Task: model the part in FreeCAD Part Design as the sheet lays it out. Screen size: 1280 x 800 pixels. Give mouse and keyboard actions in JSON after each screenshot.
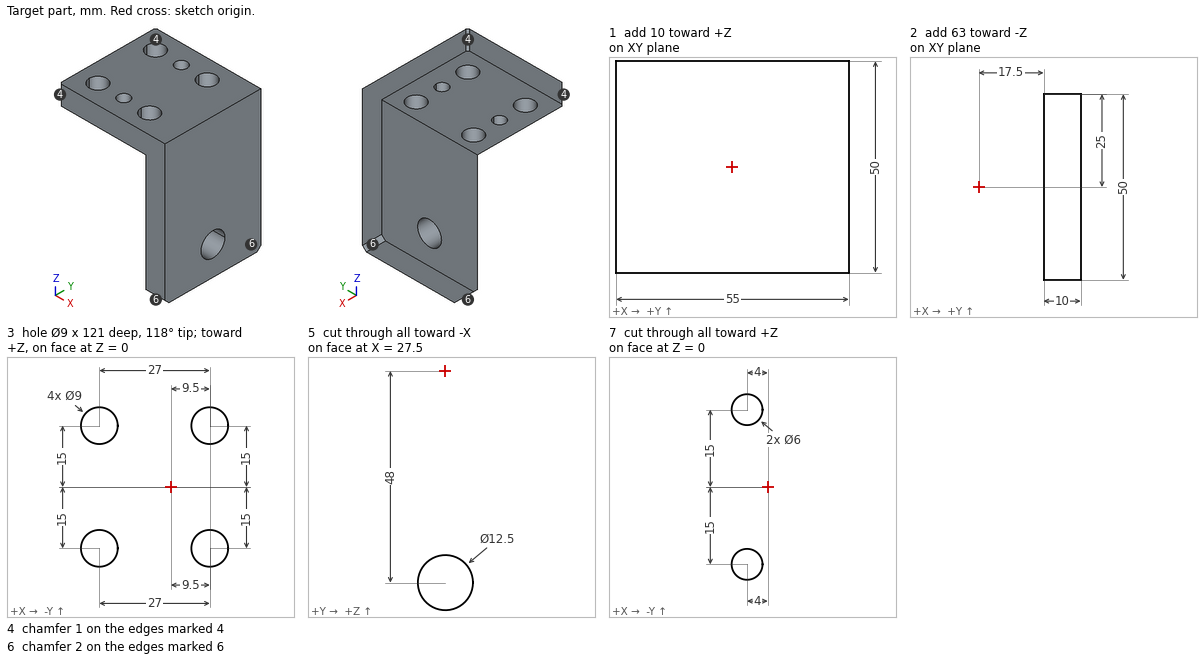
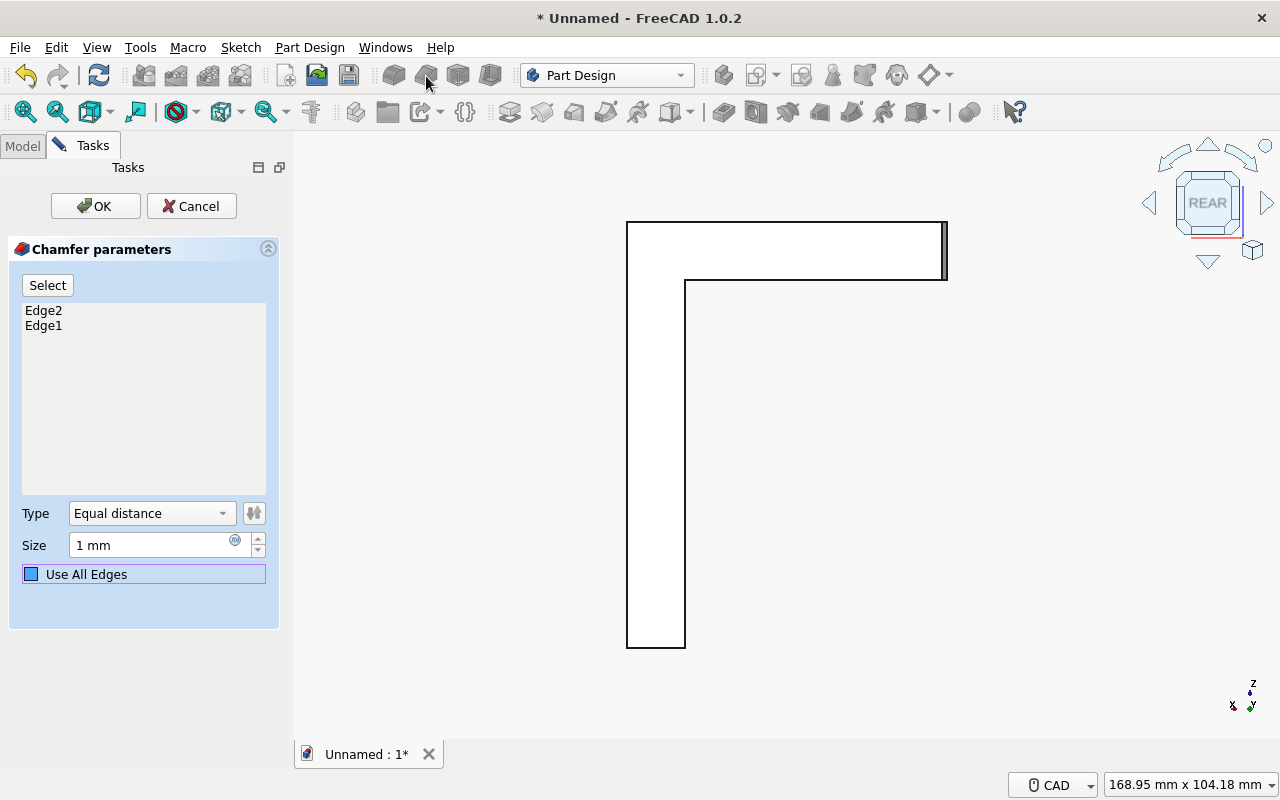
{"action": "left_click", "coordinate": [96, 206]}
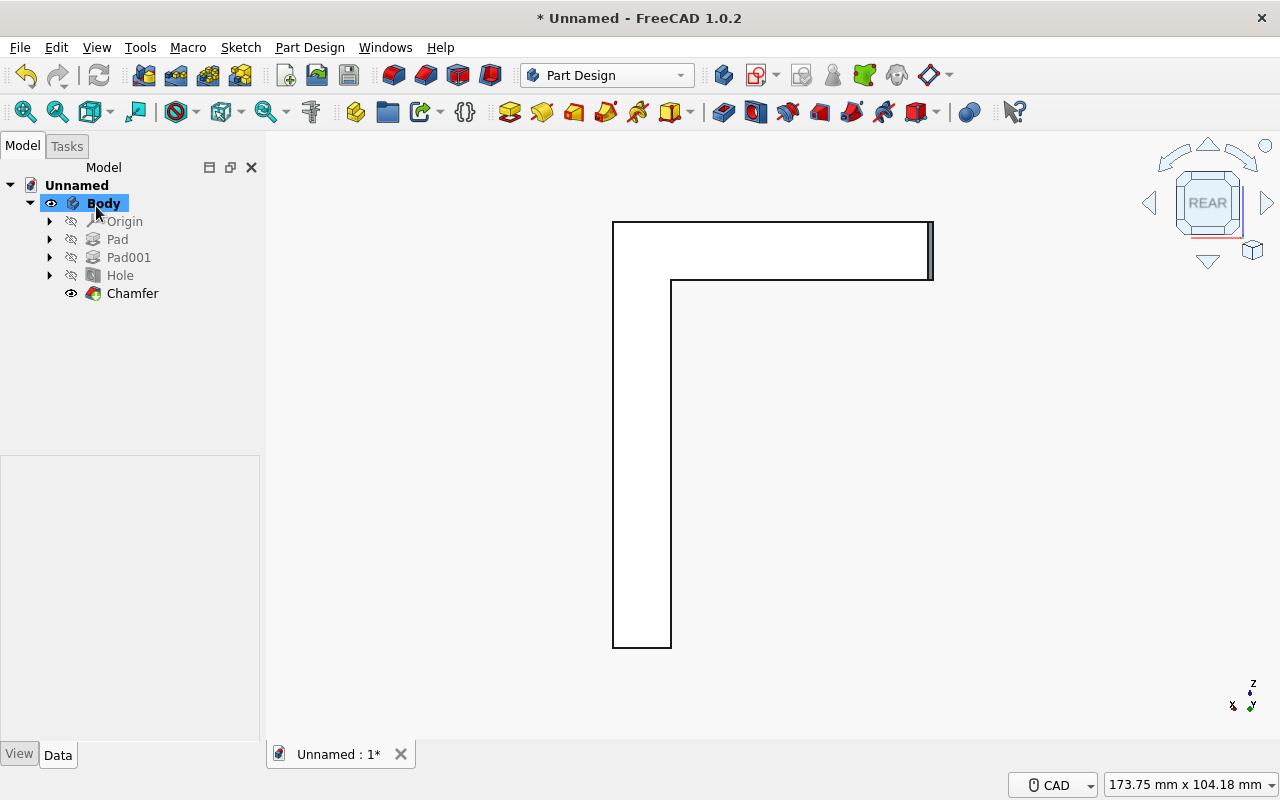
{"action": "key", "text": "0"}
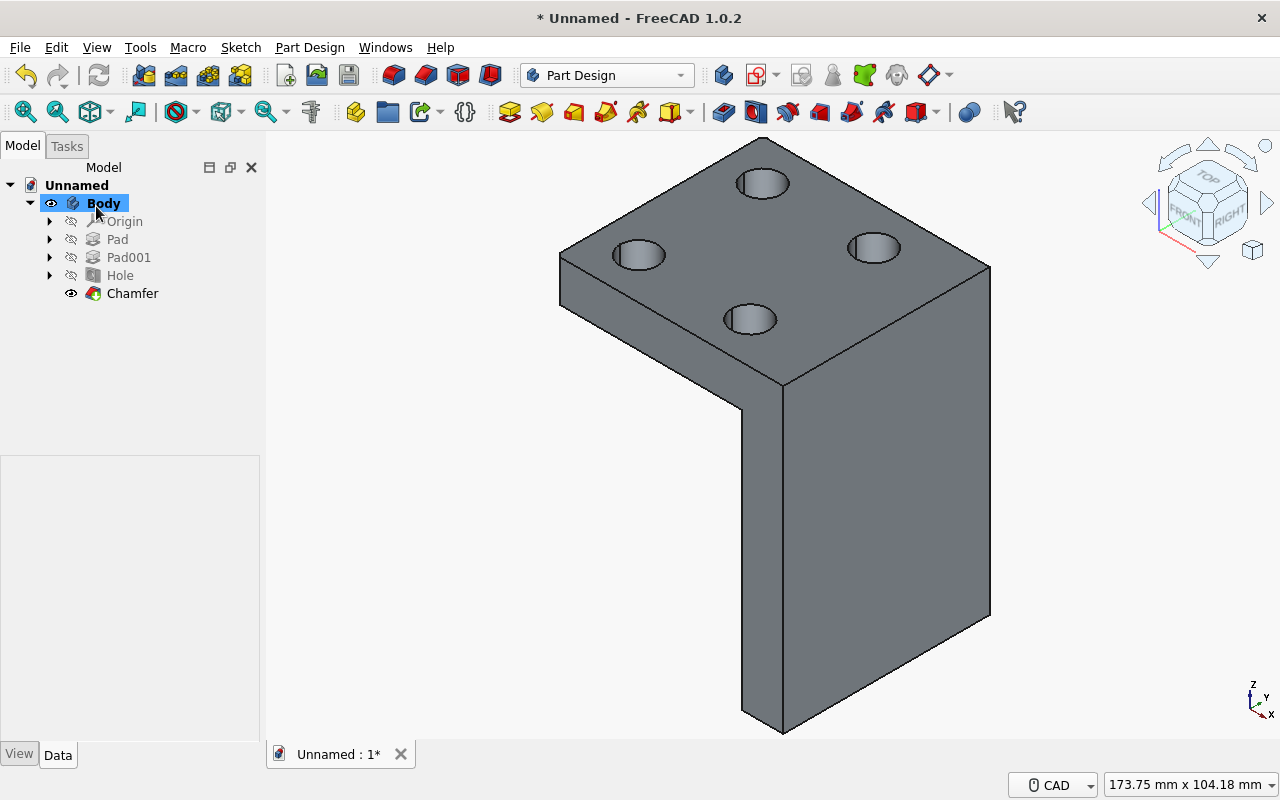
{"action": "left_click", "coordinate": [886, 450]}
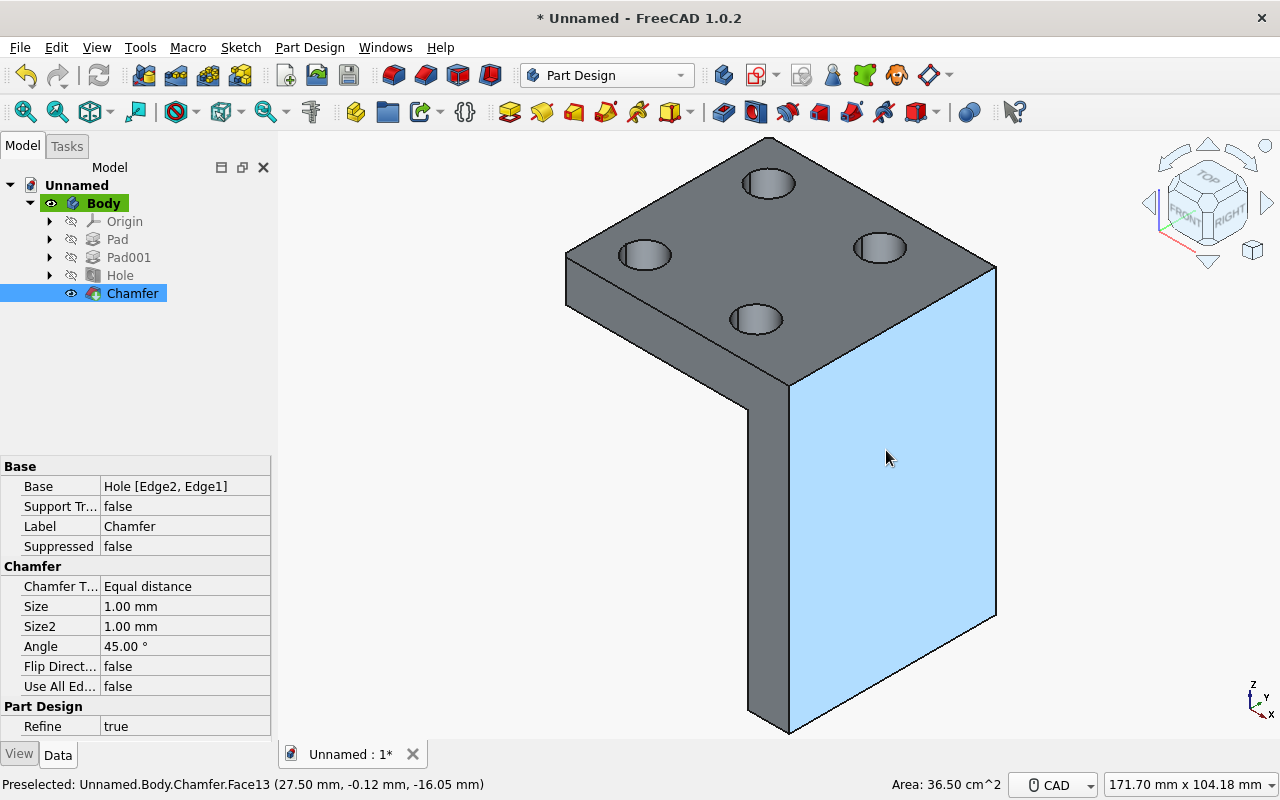
{"action": "left_click", "coordinate": [756, 76]}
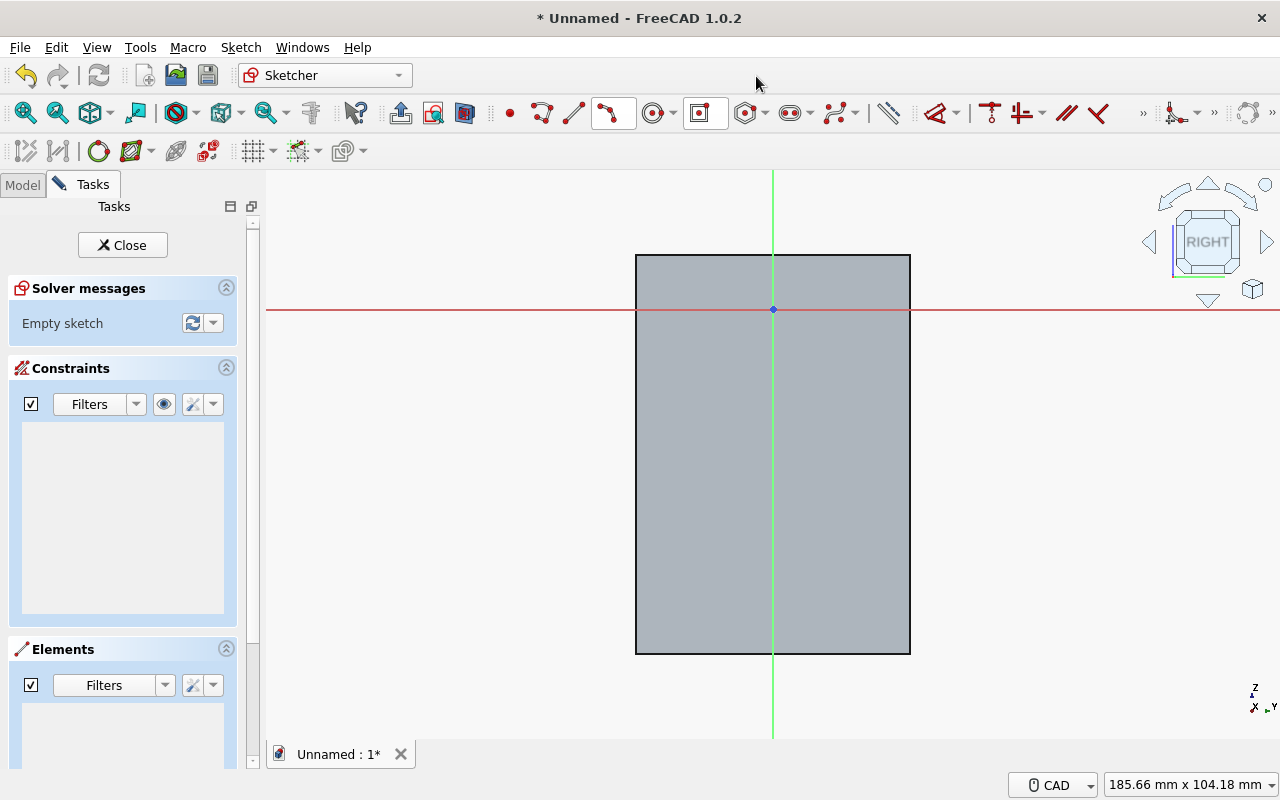
{"action": "scroll", "coordinate": [790, 602], "scroll_direction": "up", "scroll_amount": 8}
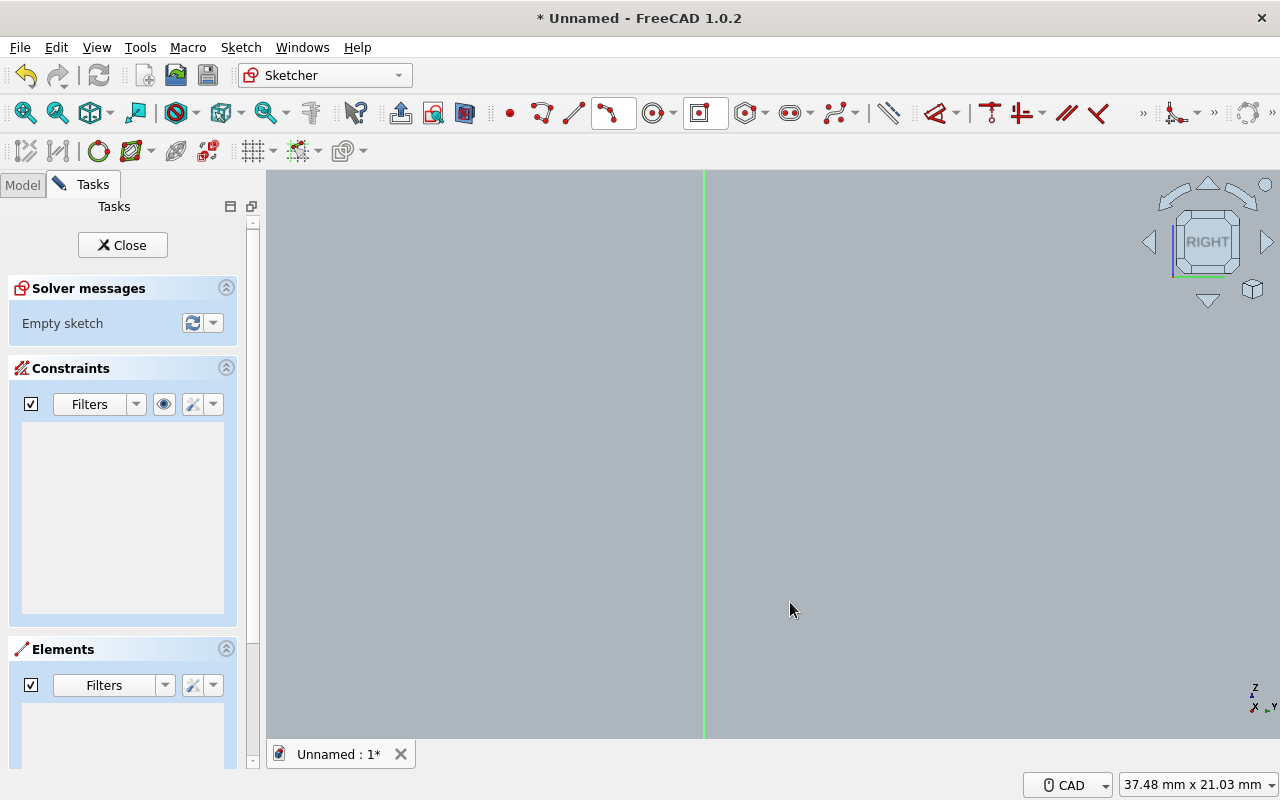
{"action": "left_click", "coordinate": [654, 114]}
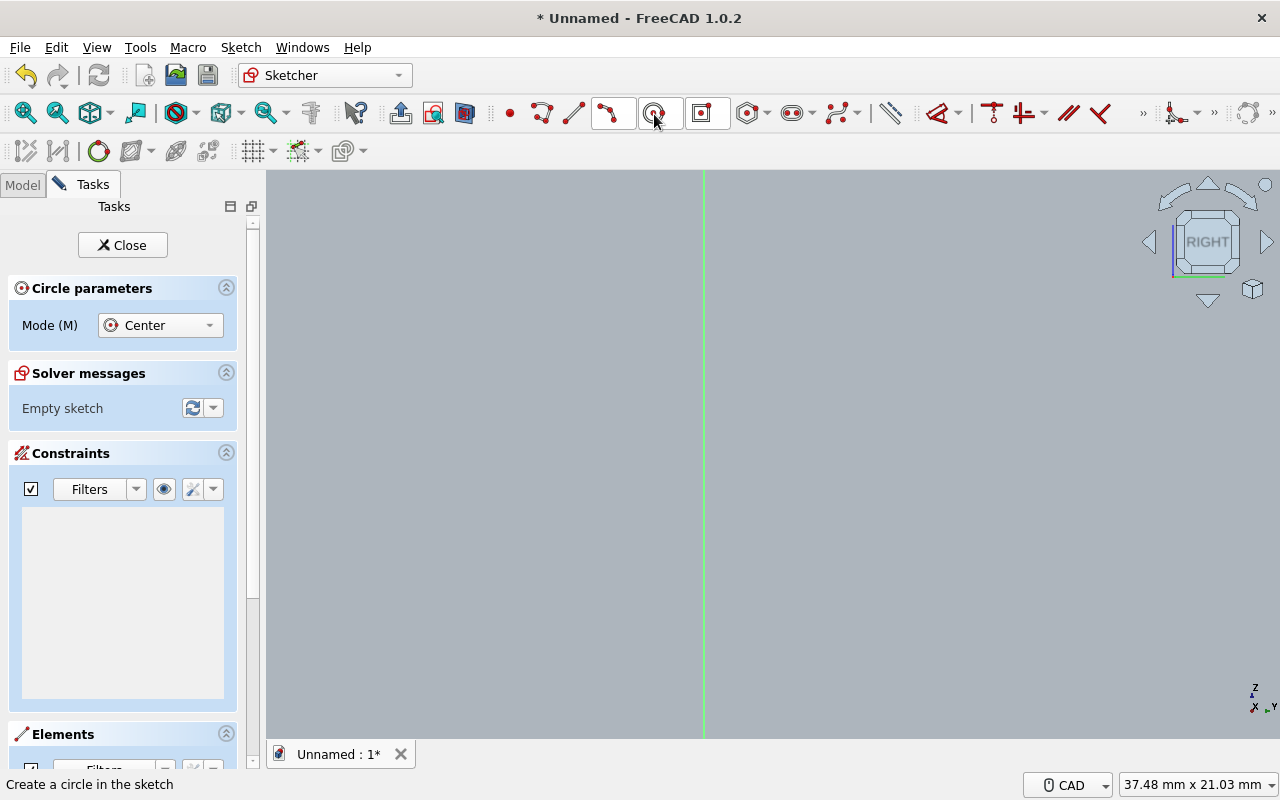
{"action": "left_click", "coordinate": [704, 450]}
{"action": "left_click", "coordinate": [823, 330]}
{"action": "key", "text": "Escape"}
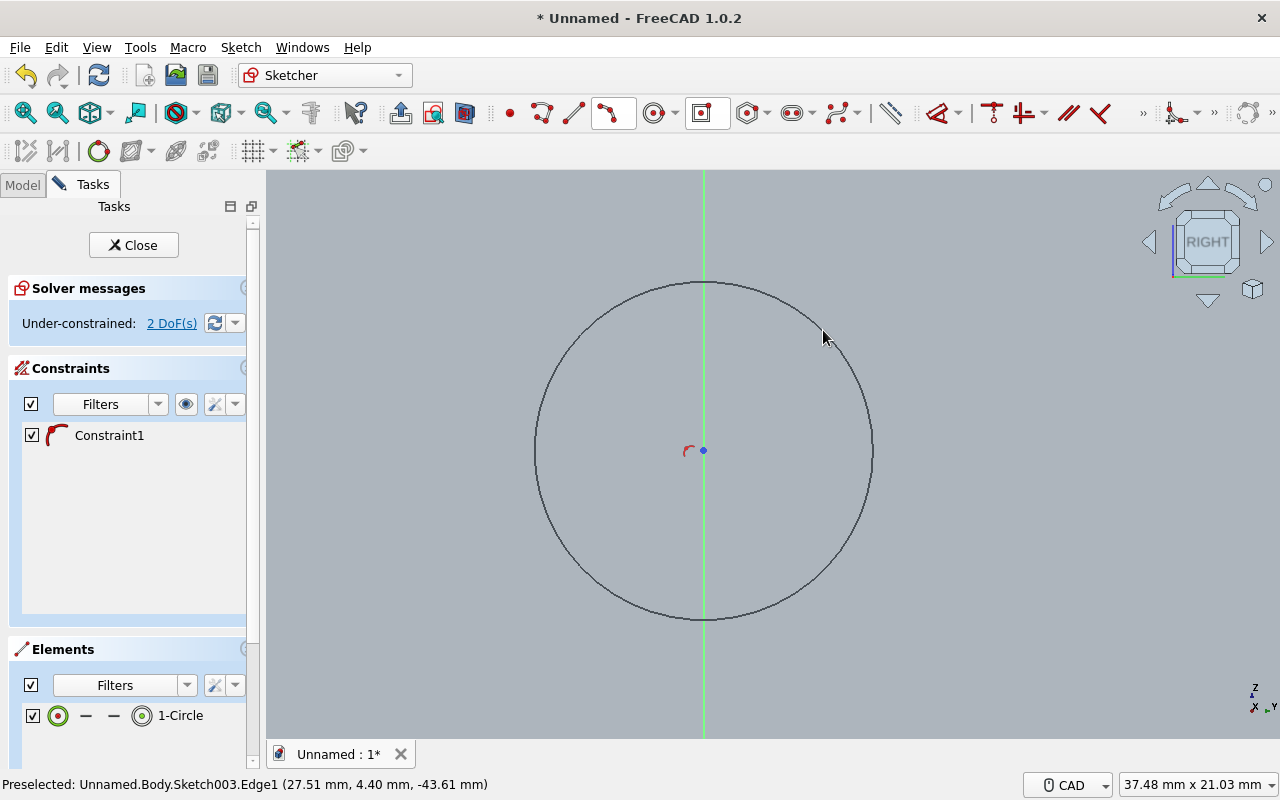
{"action": "key", "text": "d"}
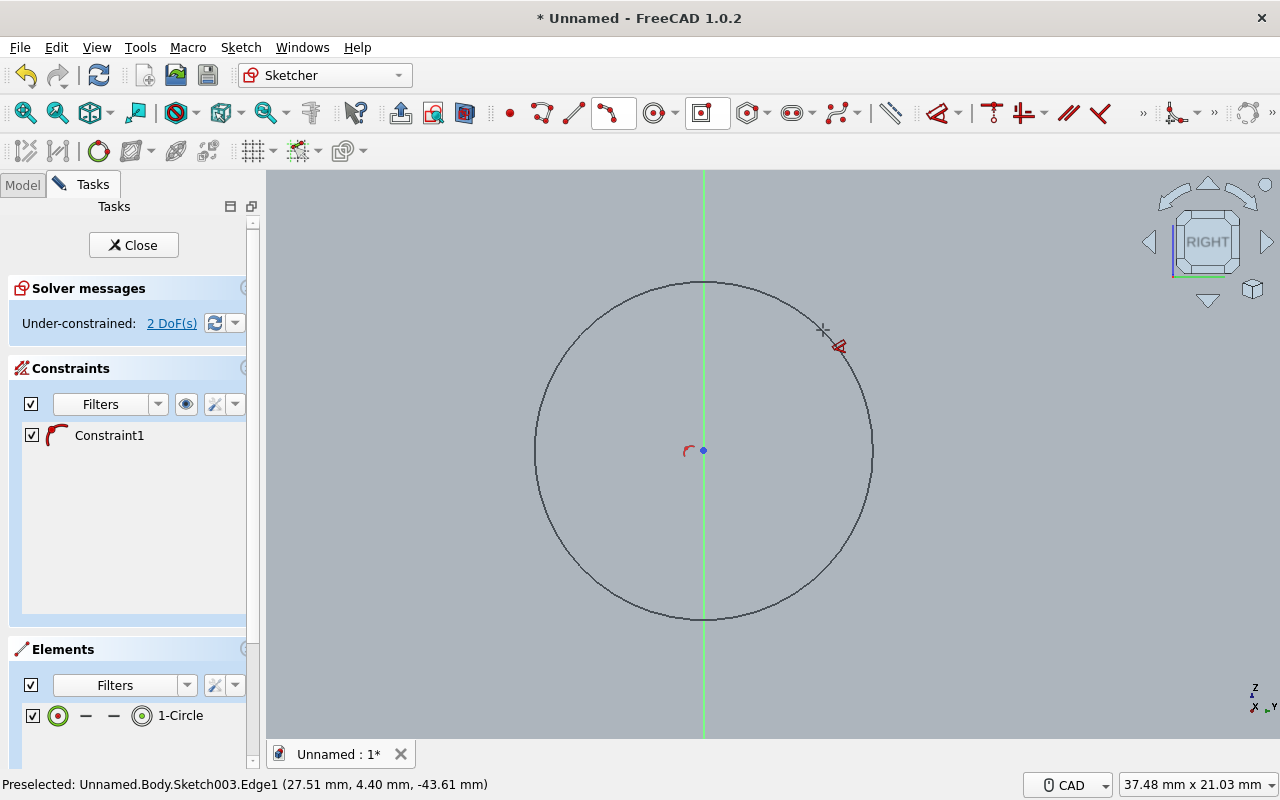
{"action": "left_click", "coordinate": [823, 331]}
{"action": "left_click", "coordinate": [846, 308]}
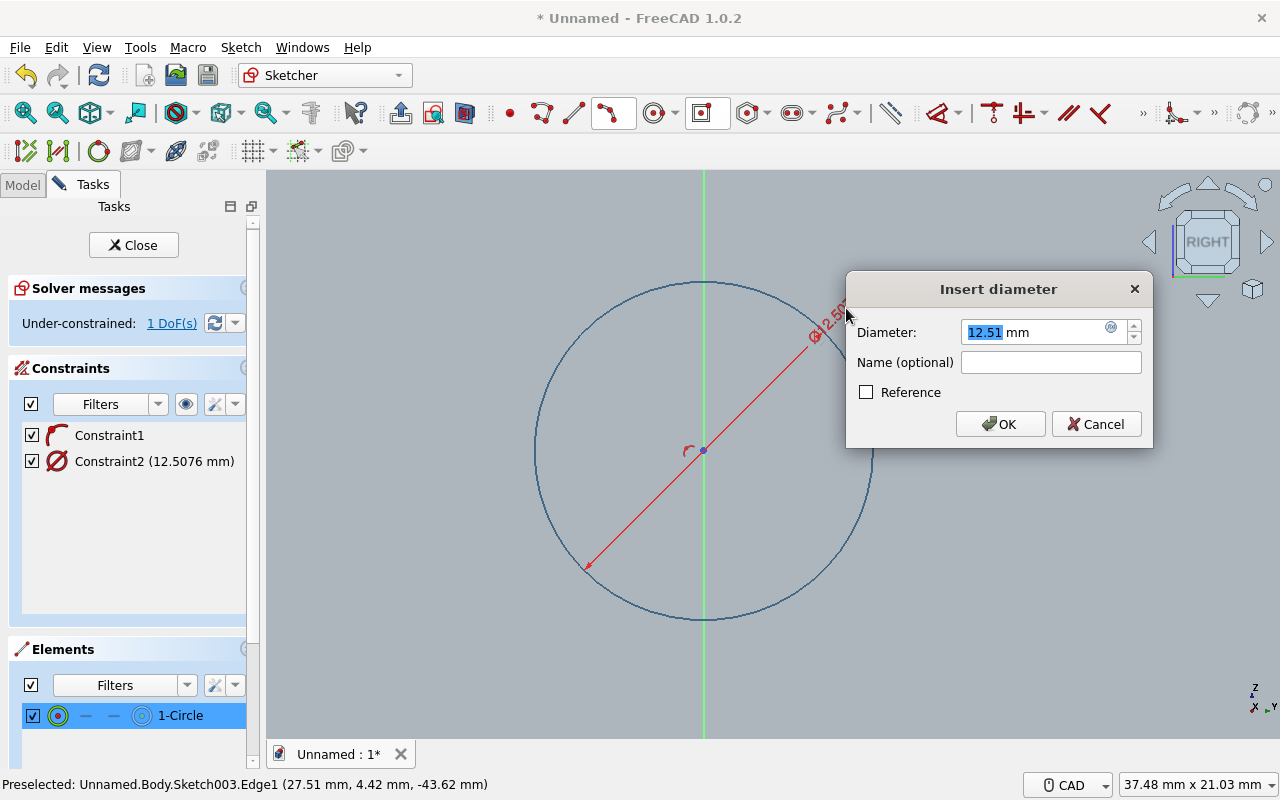
{"action": "type", "text": "12.5"}
{"action": "key", "text": "Return"}